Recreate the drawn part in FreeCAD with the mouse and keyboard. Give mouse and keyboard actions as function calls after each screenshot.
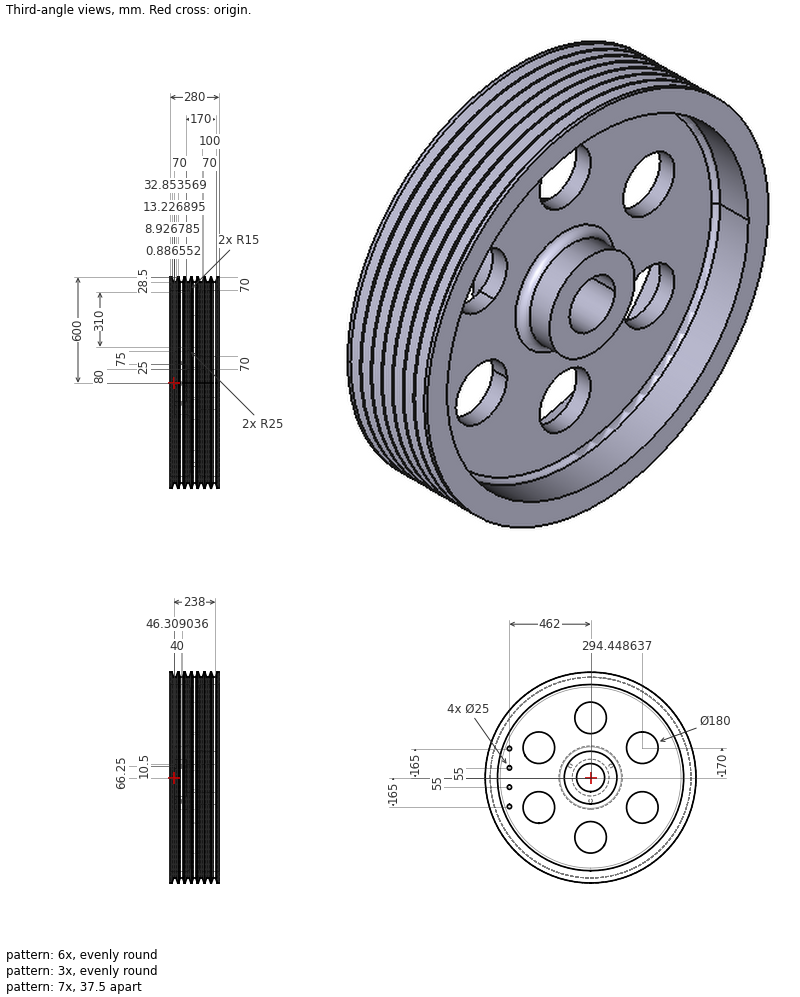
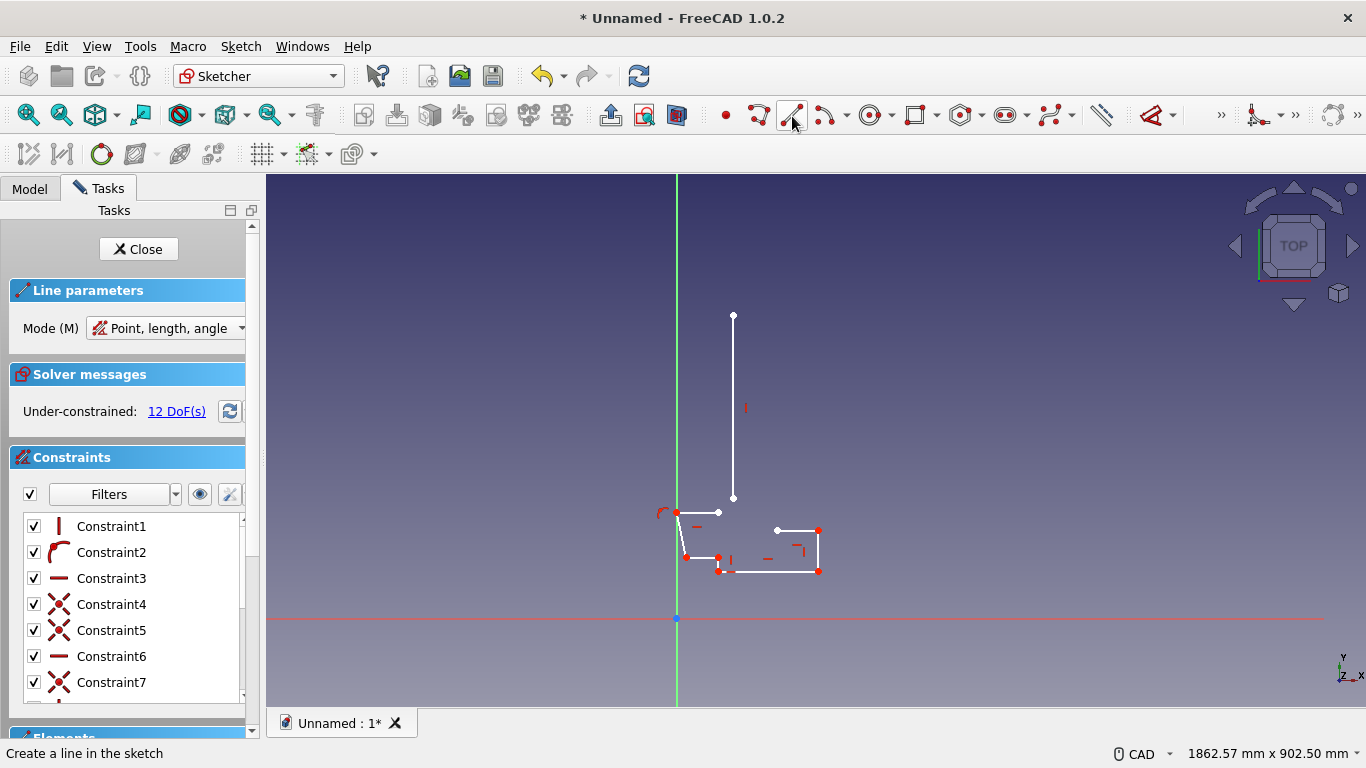
click(762, 515)
click(762, 315)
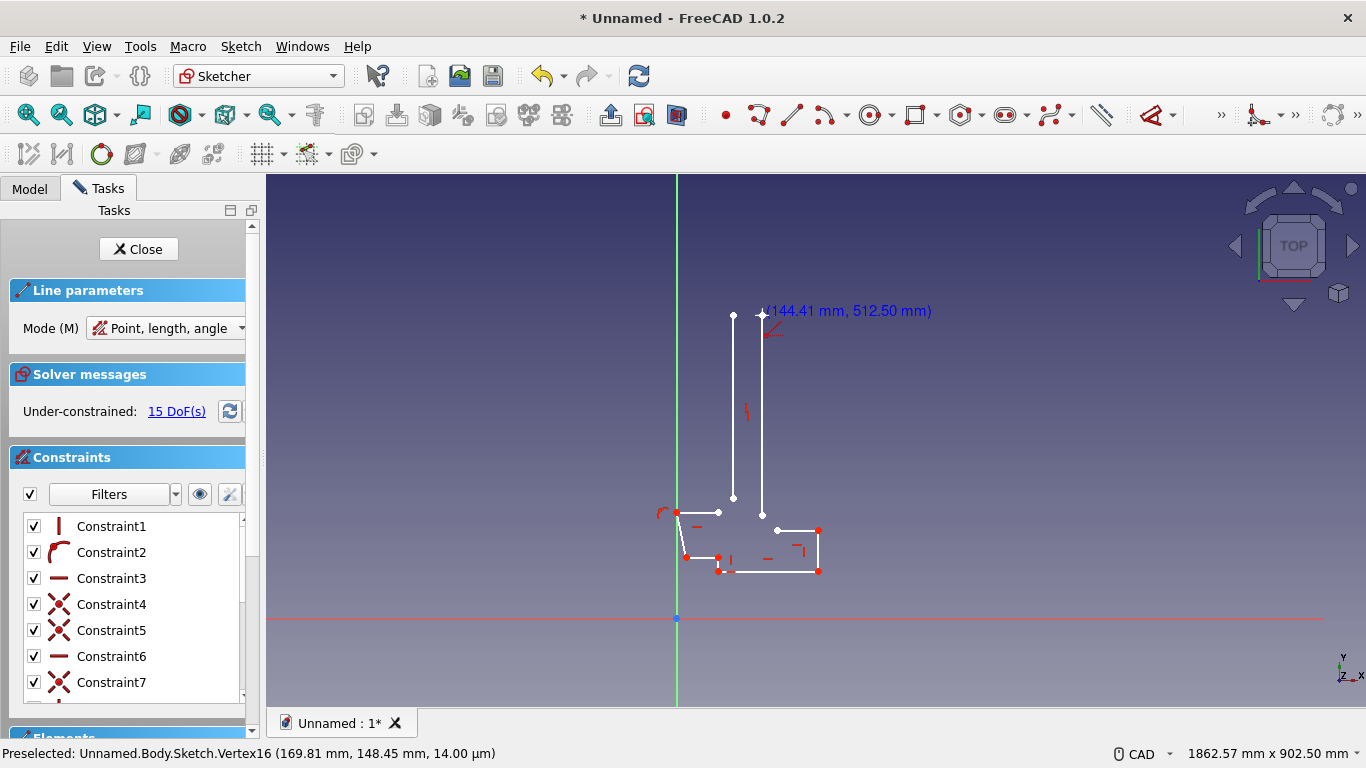
click(759, 116)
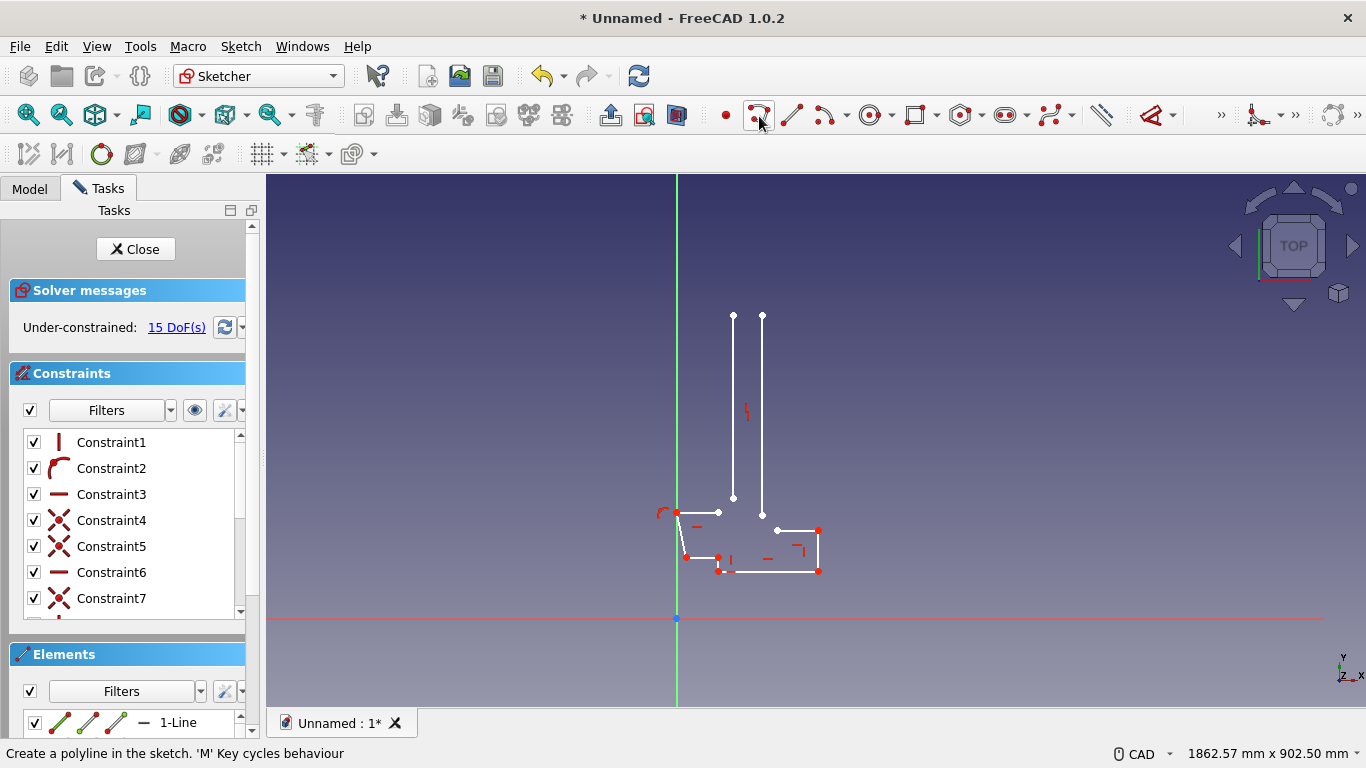
scroll(771, 306, up, 2)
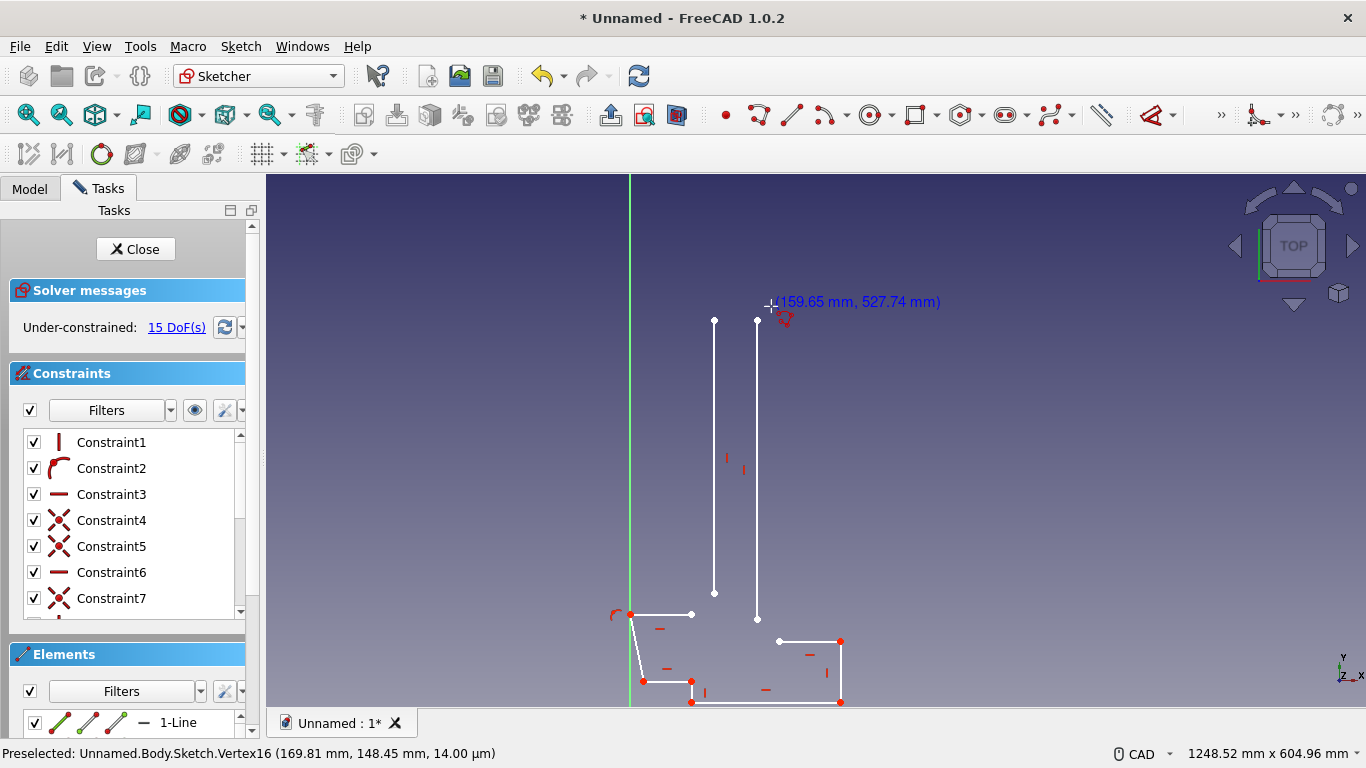
click(771, 305)
click(859, 305)
click(859, 244)
click(612, 244)
click(612, 305)
click(701, 305)
right_click(701, 305)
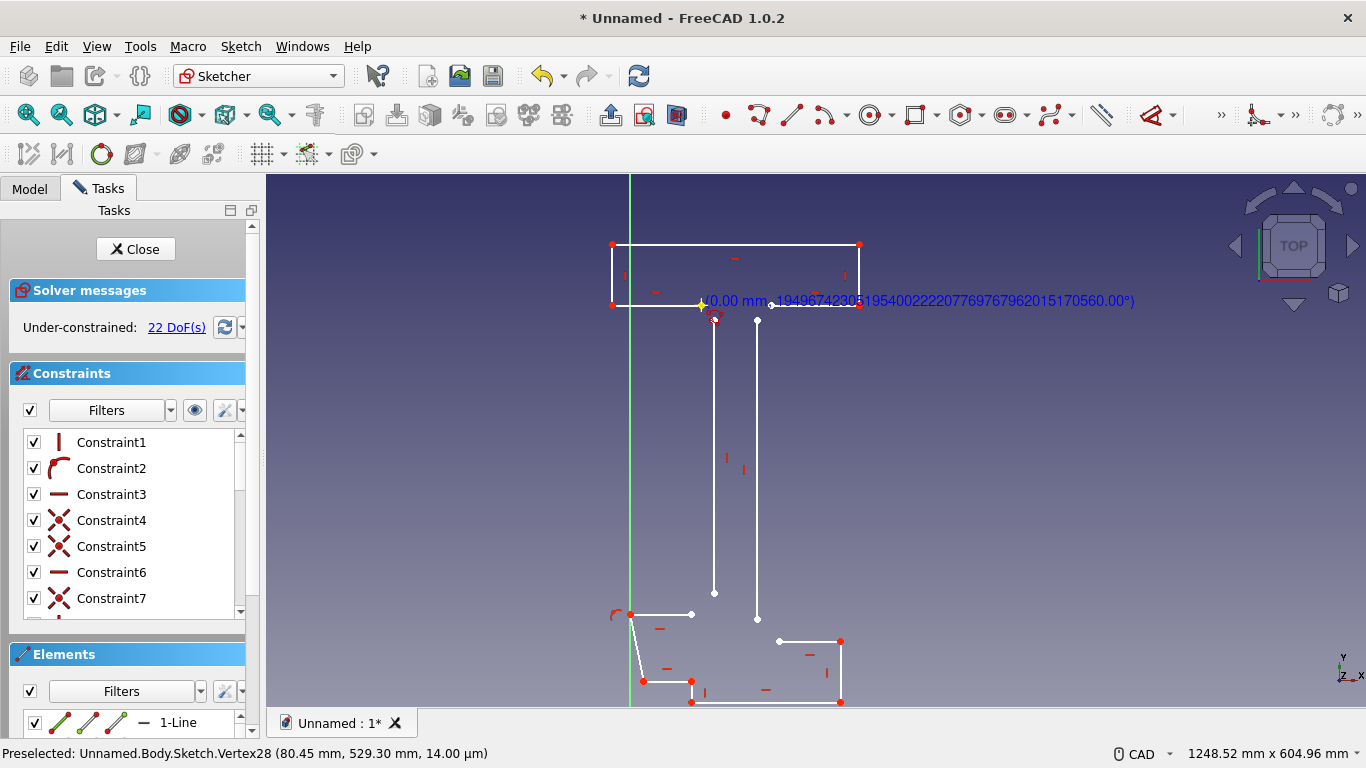
click(846, 116)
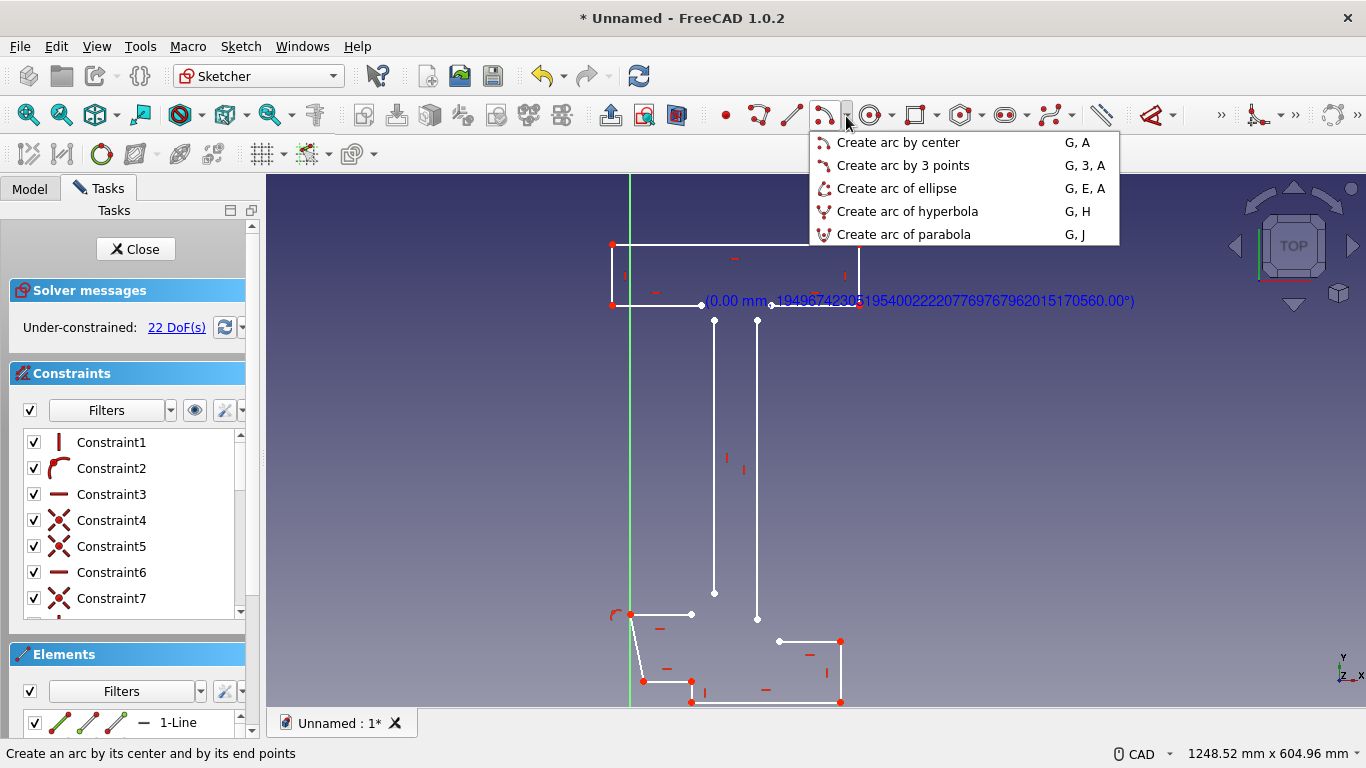
click(964, 166)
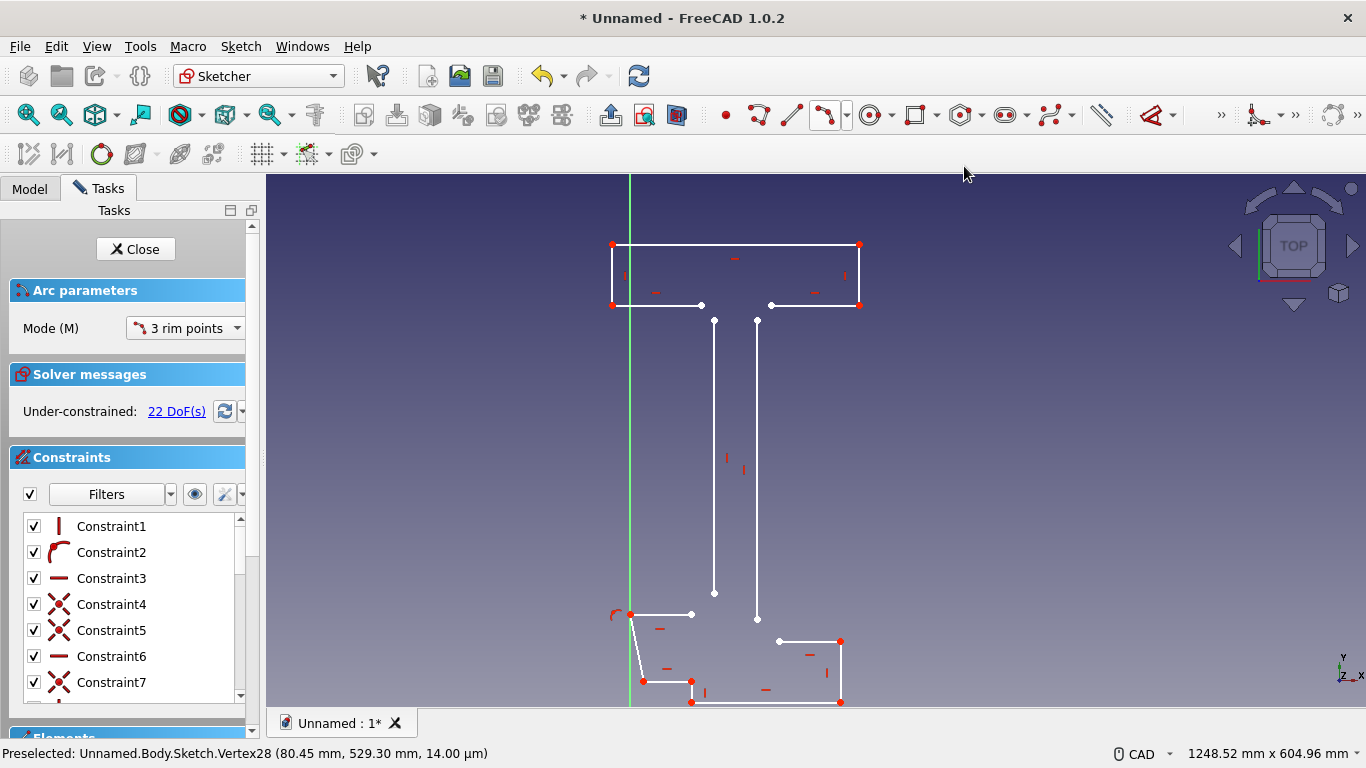
click(714, 594)
click(692, 615)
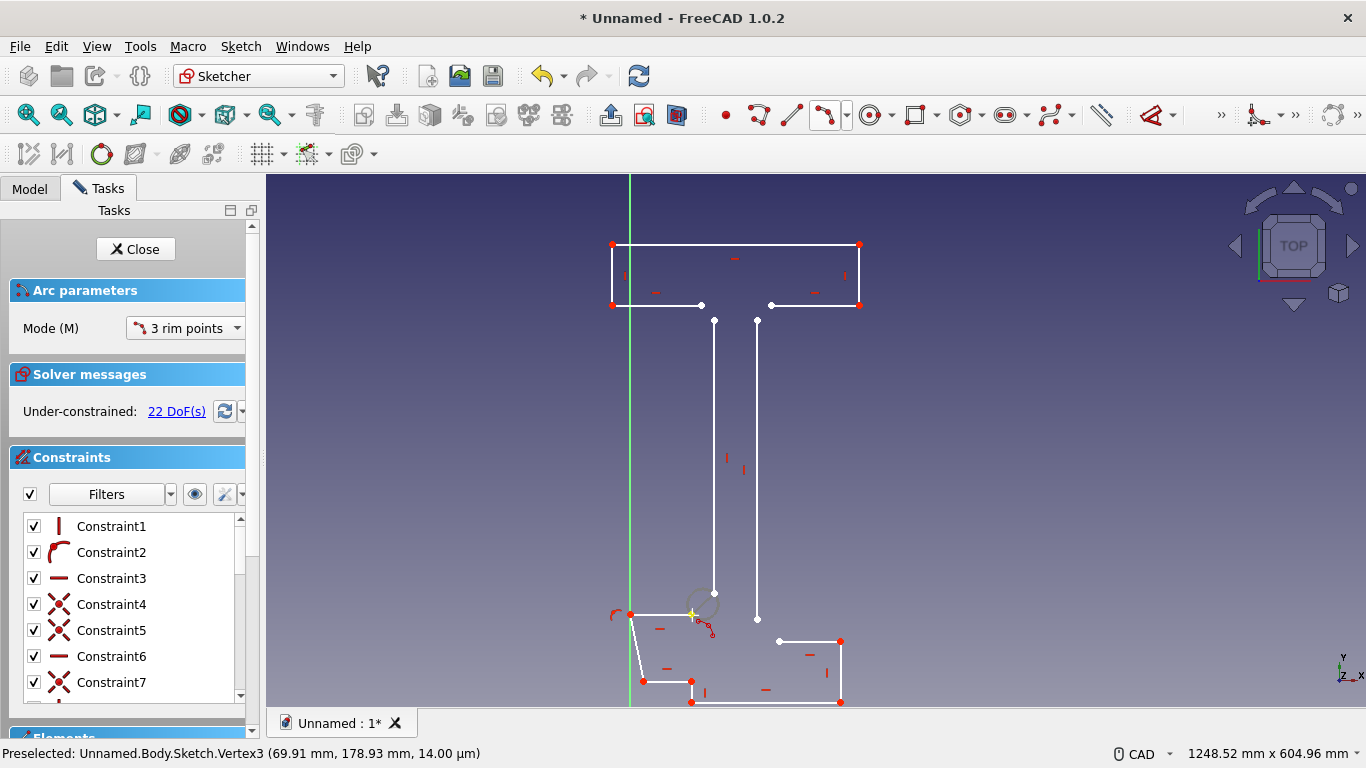
scroll(707, 607, up, 5)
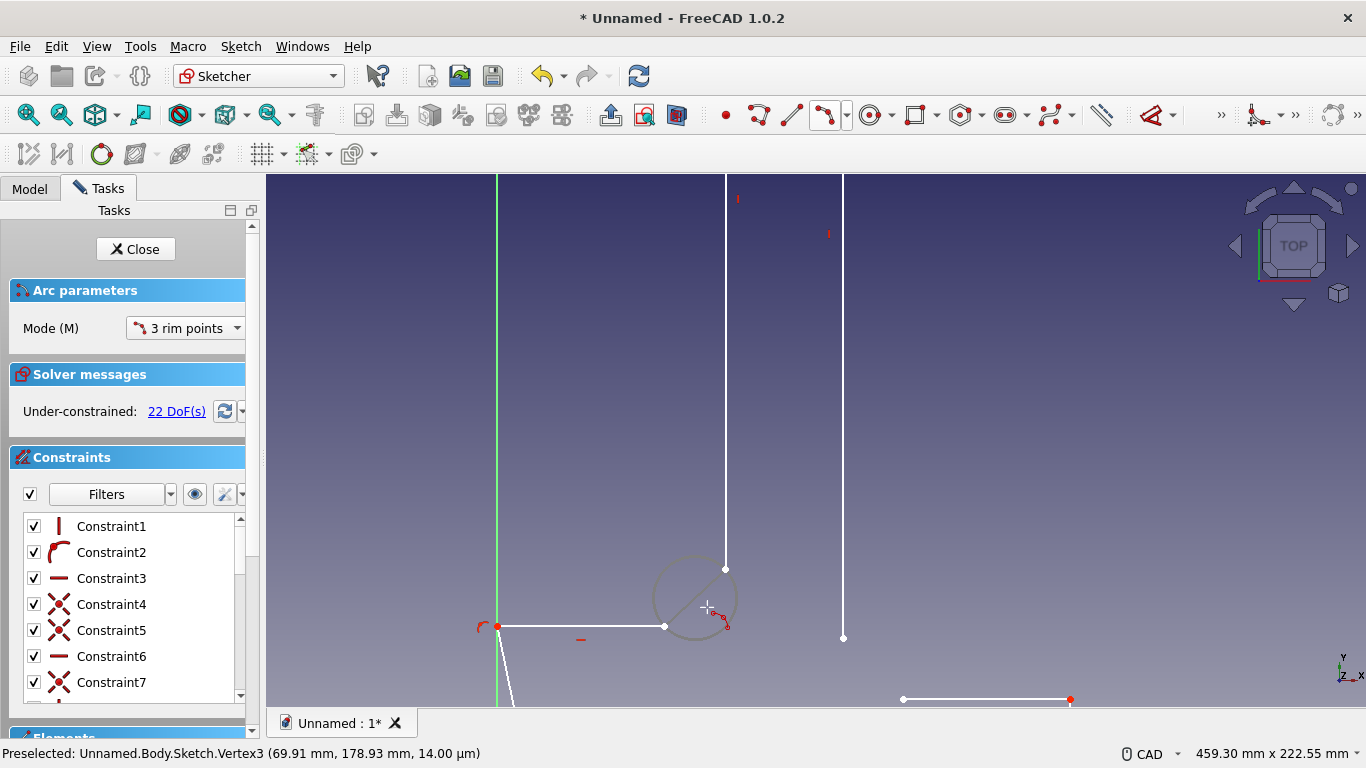
click(707, 606)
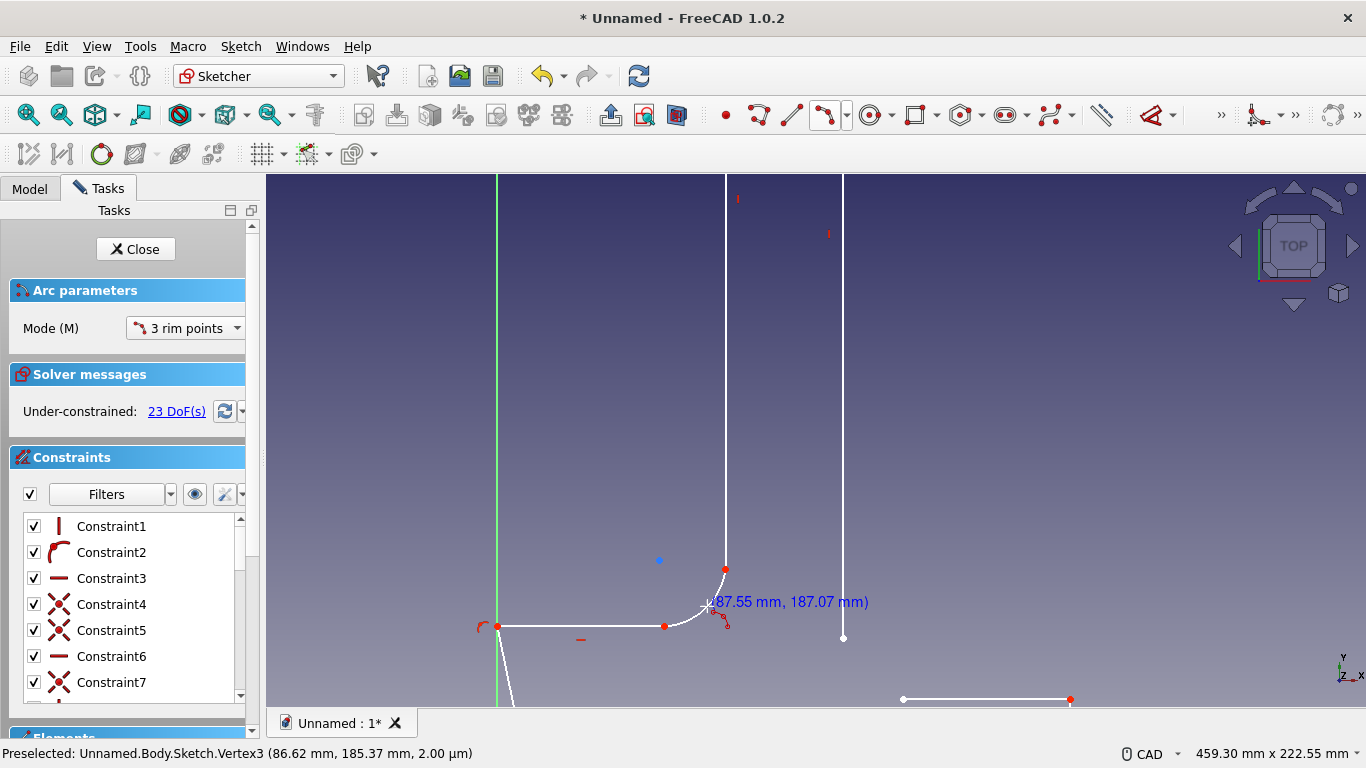
scroll(735, 475, down, 7)